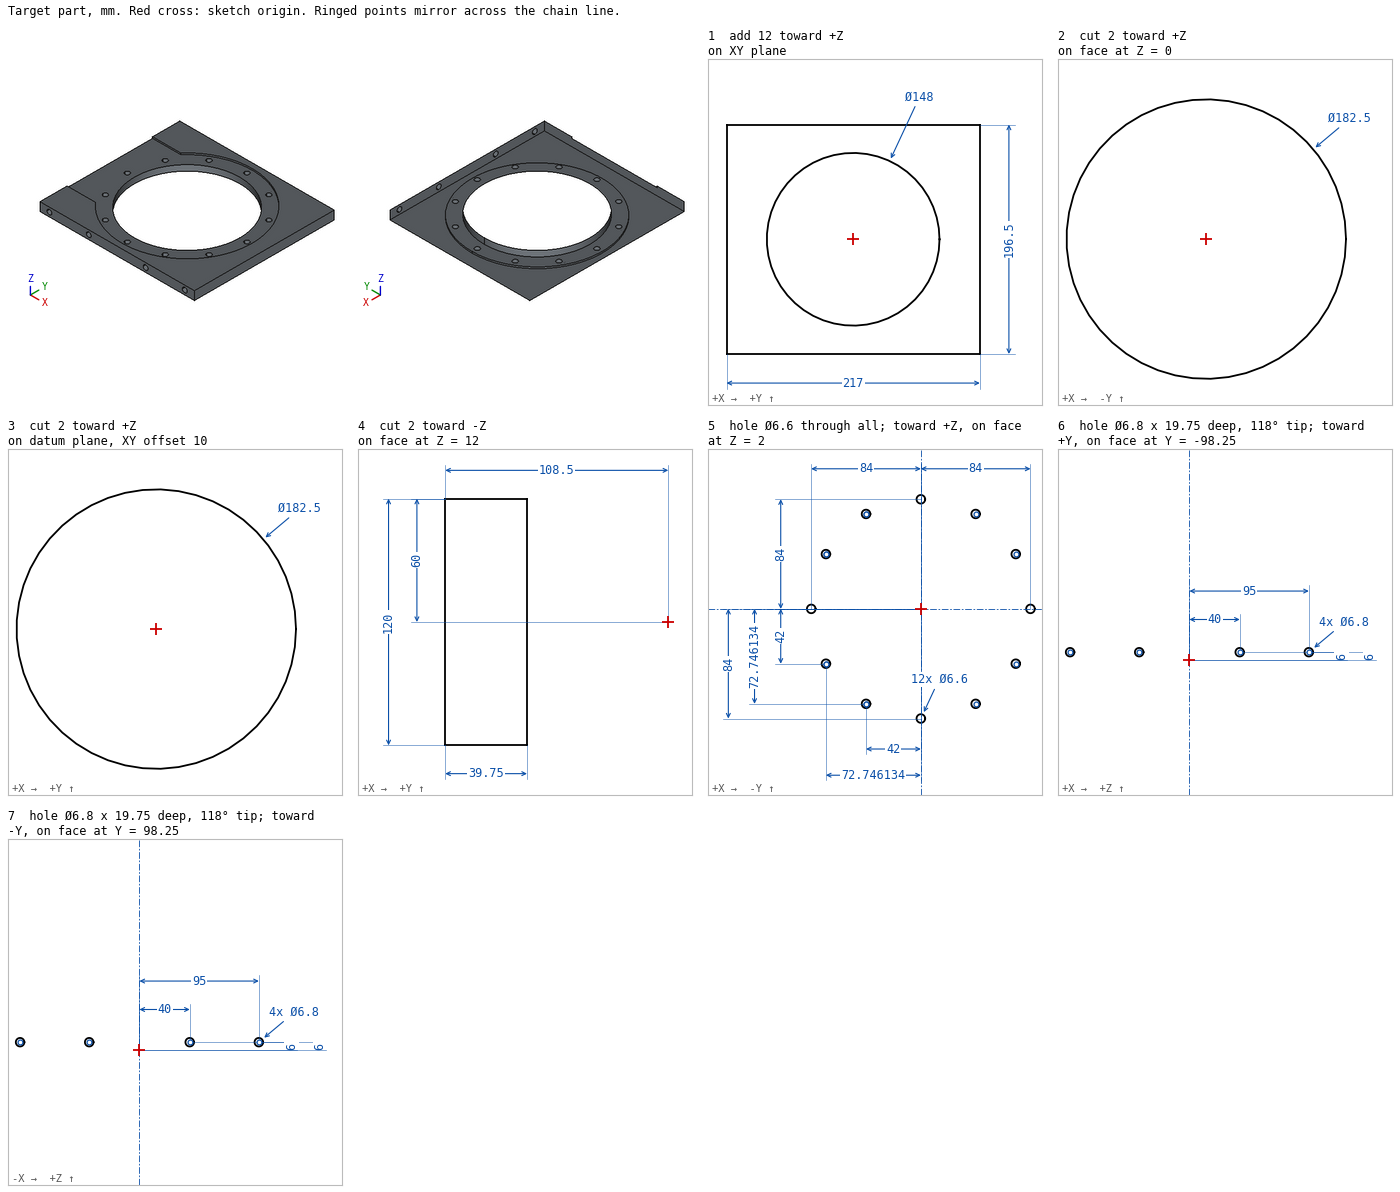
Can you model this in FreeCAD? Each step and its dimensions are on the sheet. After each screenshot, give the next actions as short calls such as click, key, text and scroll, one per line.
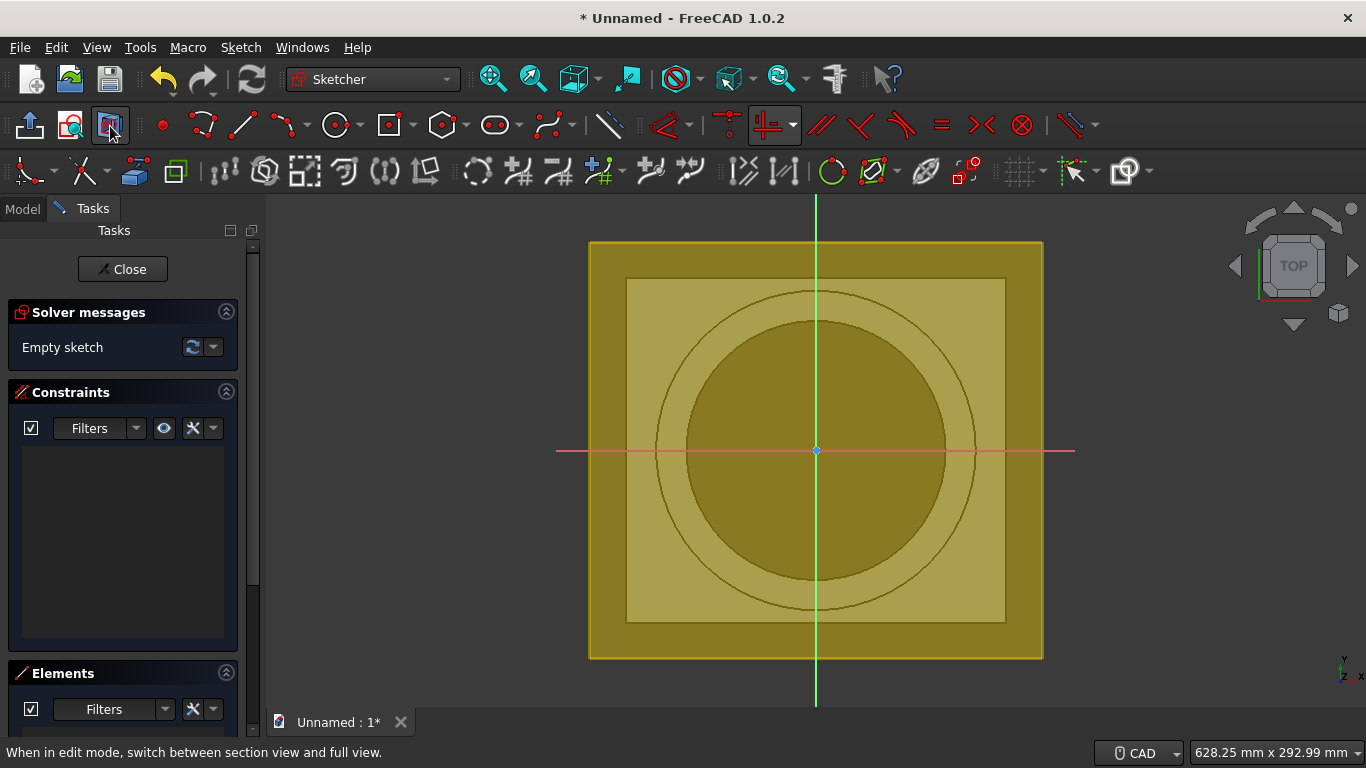
click(336, 126)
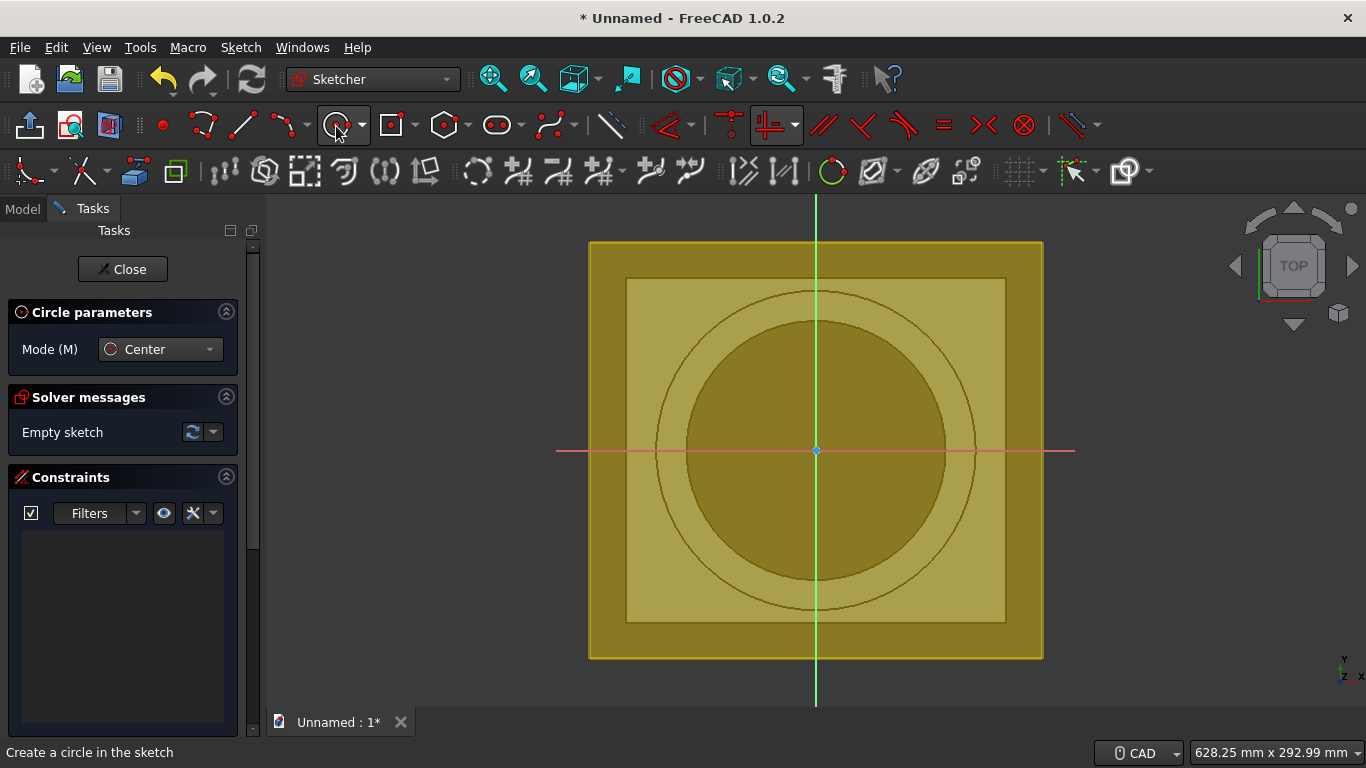
click(816, 450)
click(929, 338)
key(Escape)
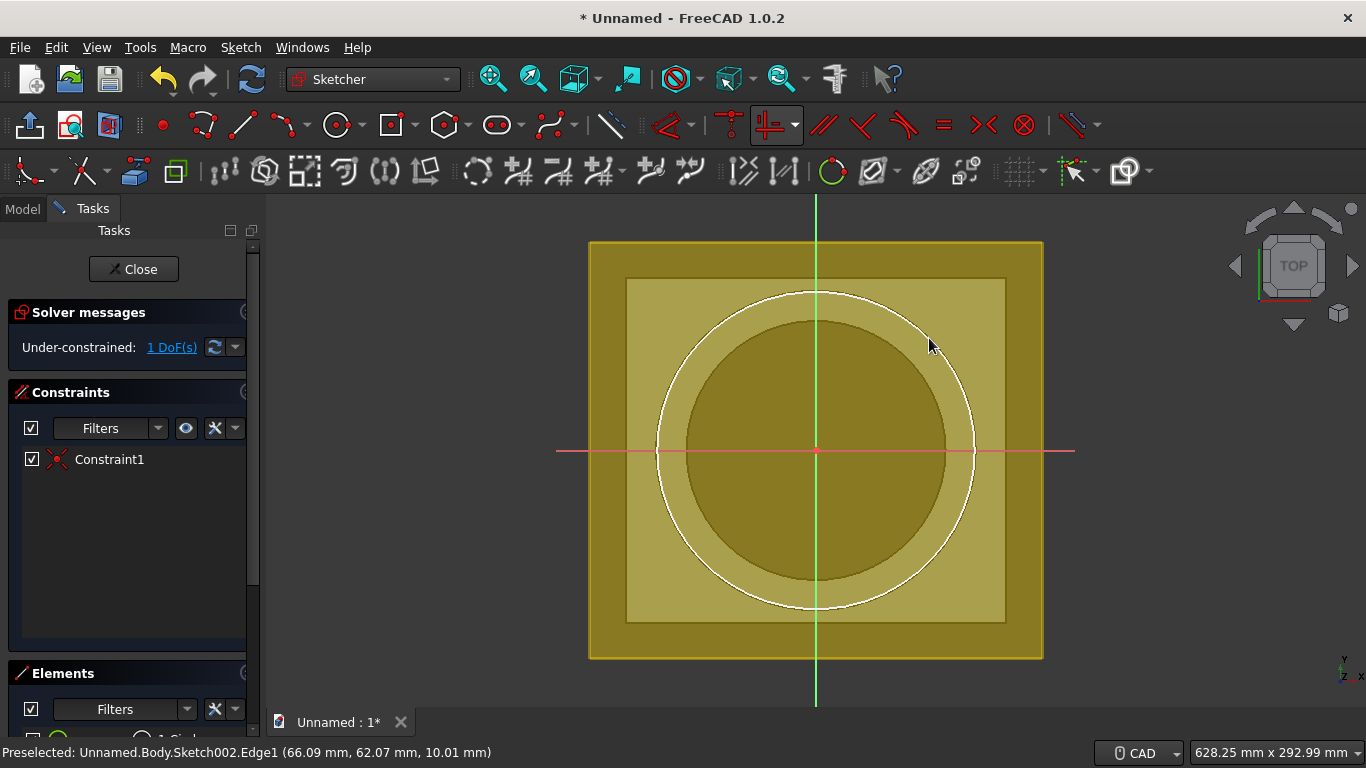
click(666, 126)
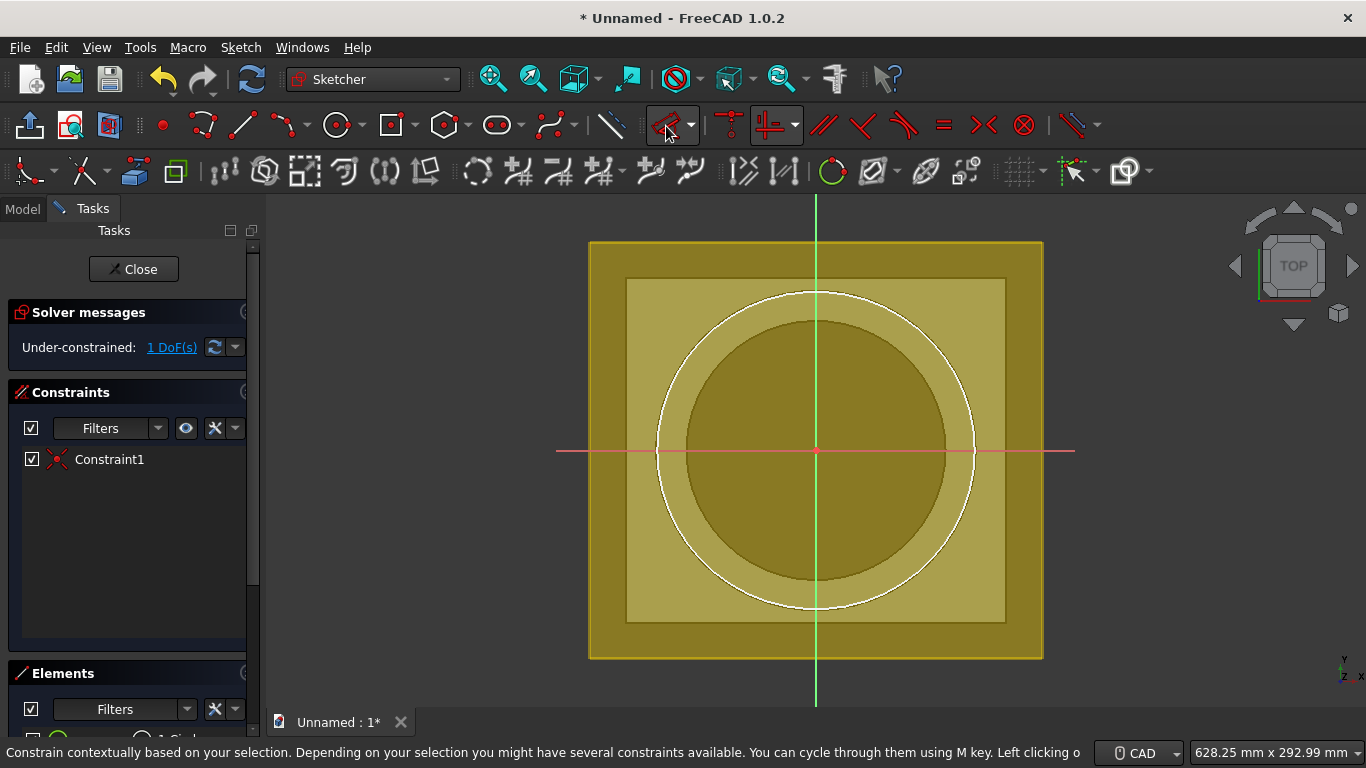
click(928, 338)
click(951, 315)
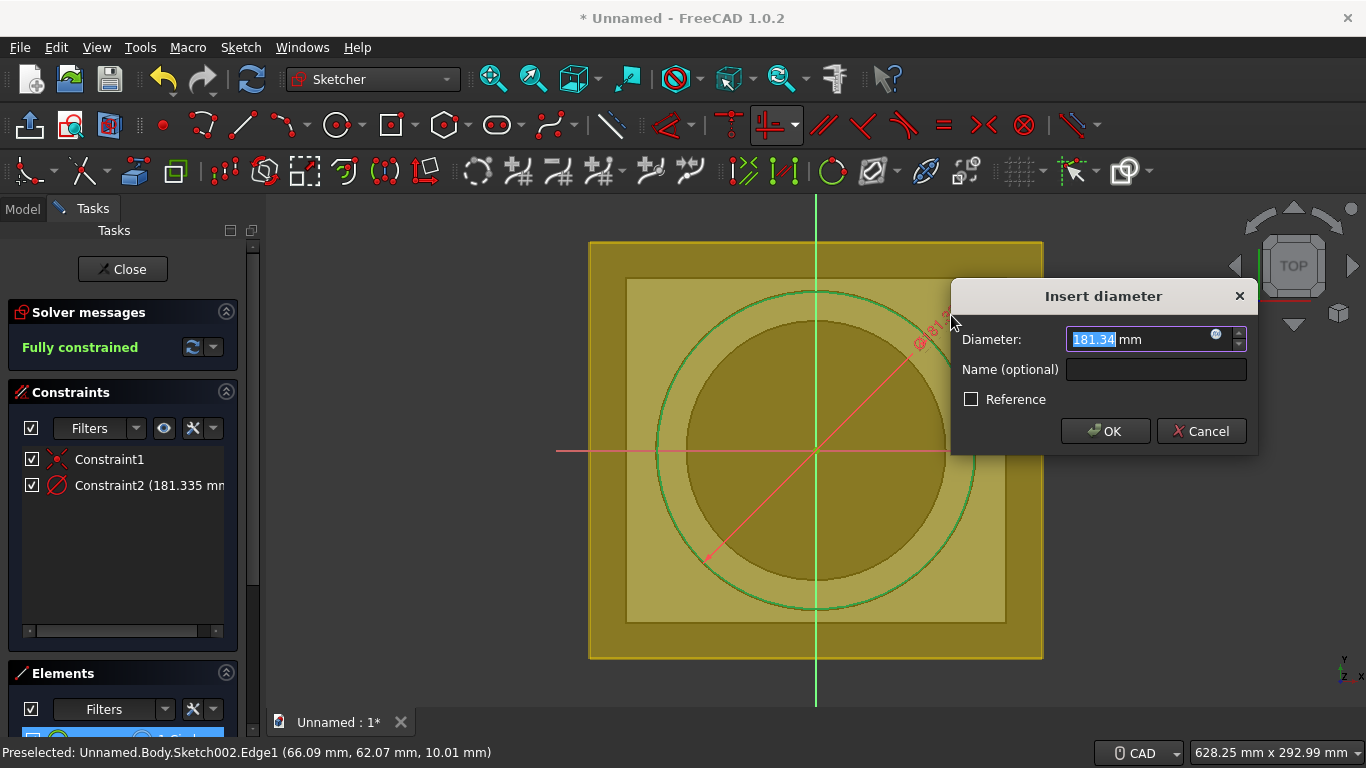
text(182.5)
key(Return)
key(Escape)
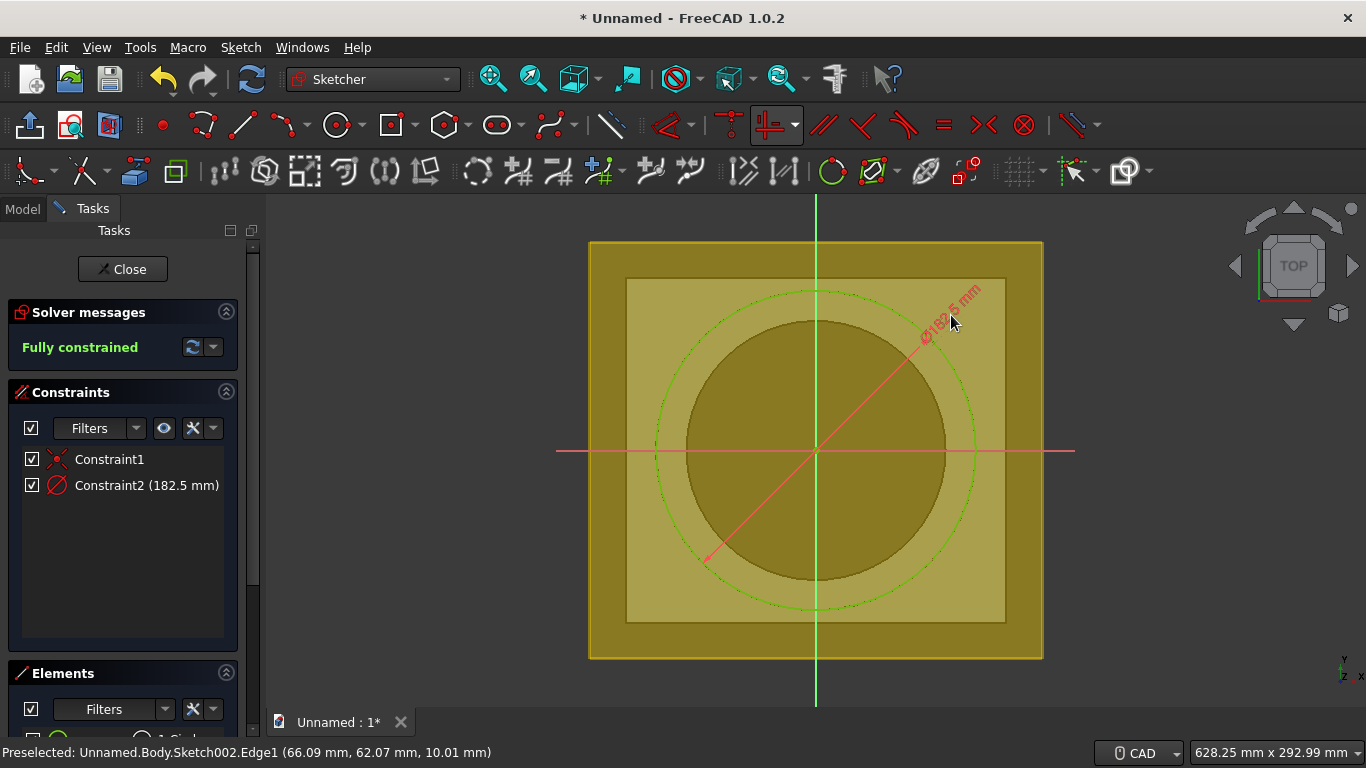
click(123, 269)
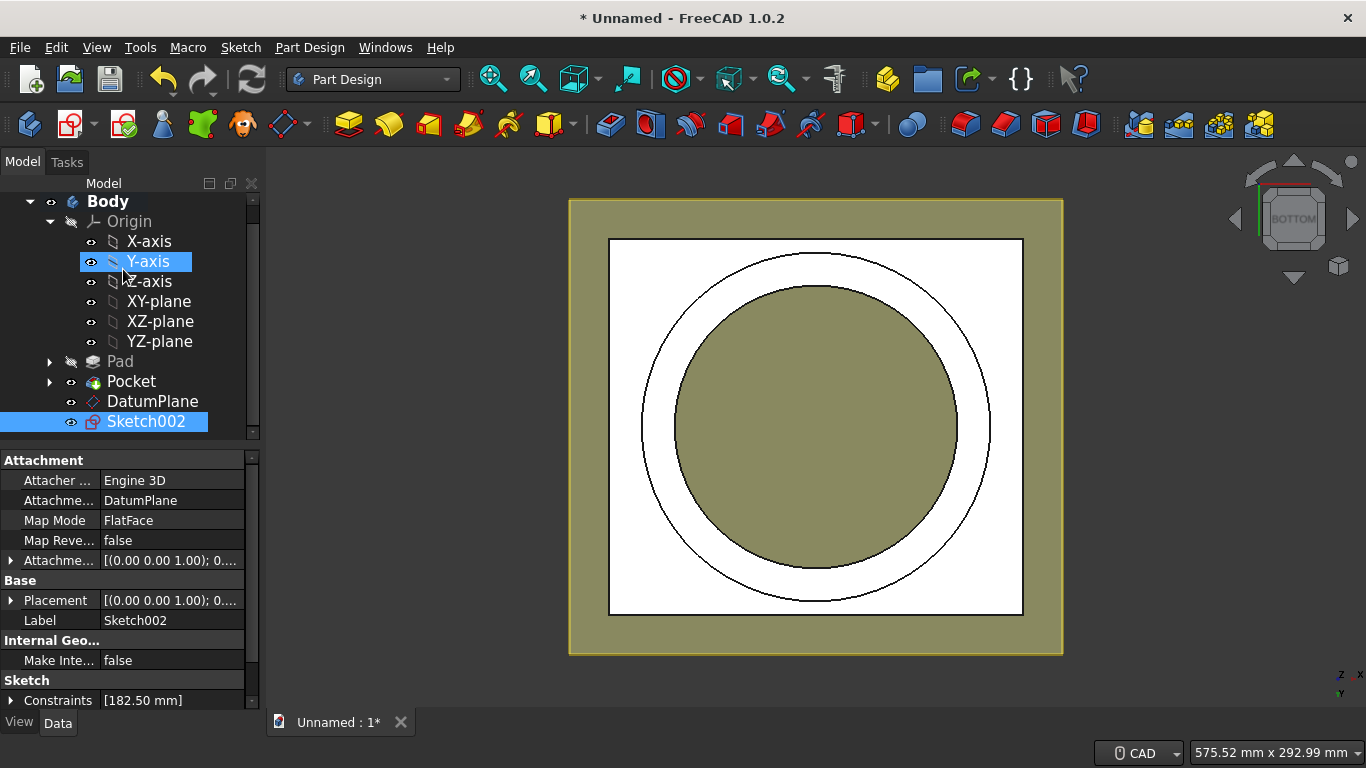
click(612, 124)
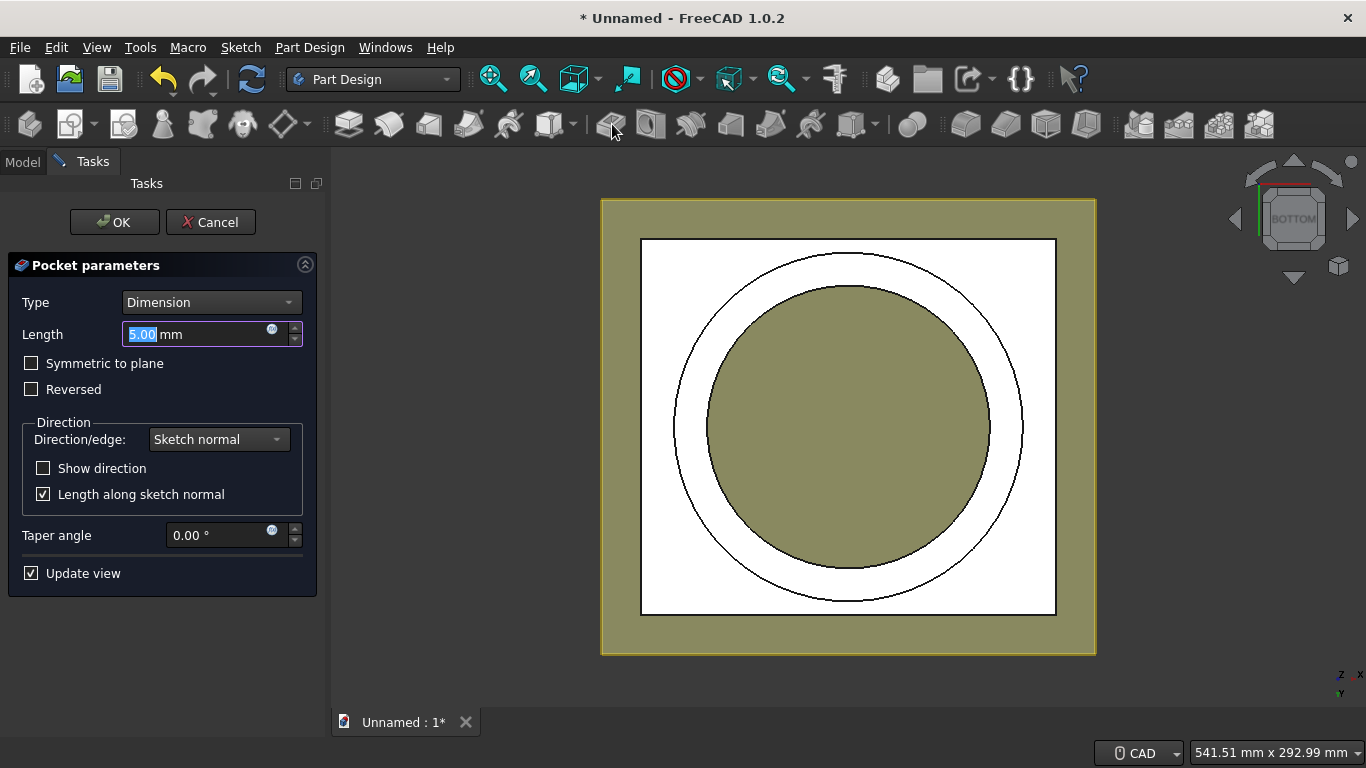
text(2)
key(Tab)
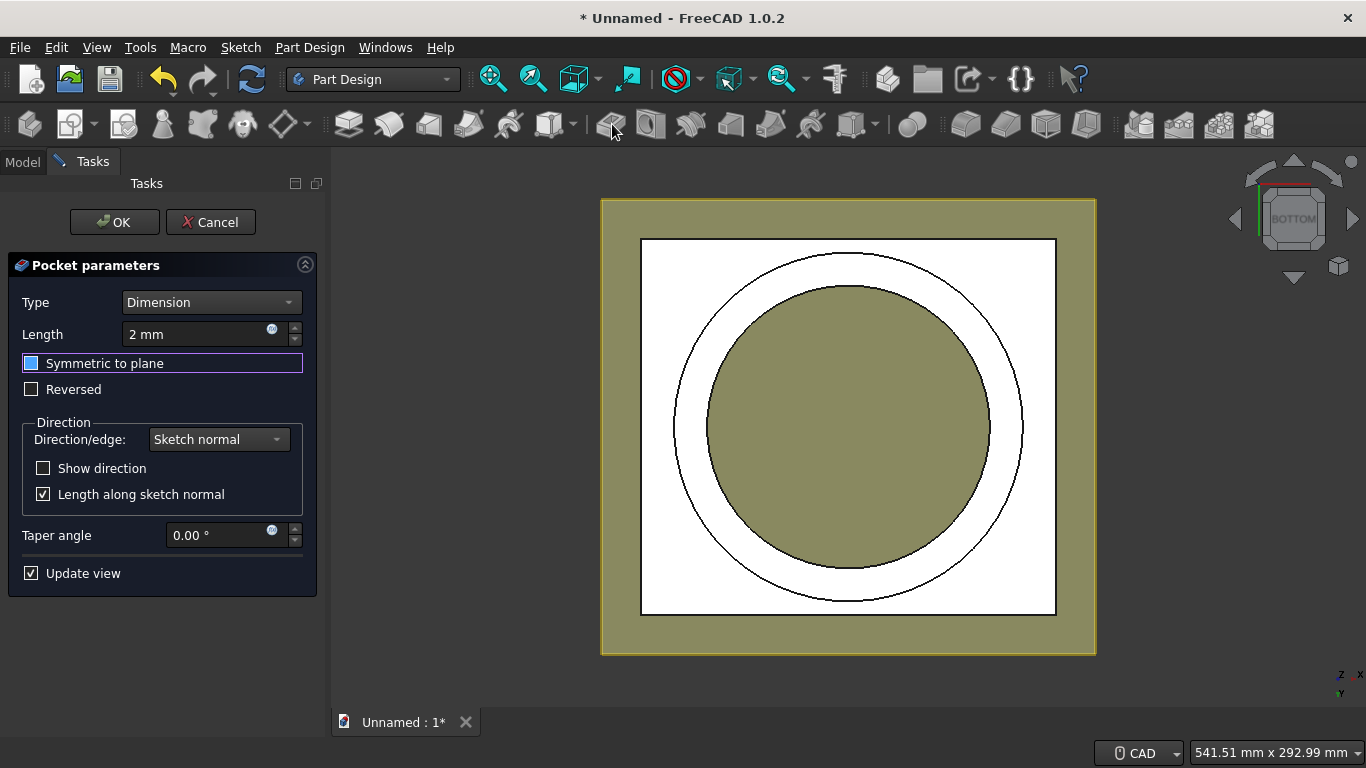
click(30, 389)